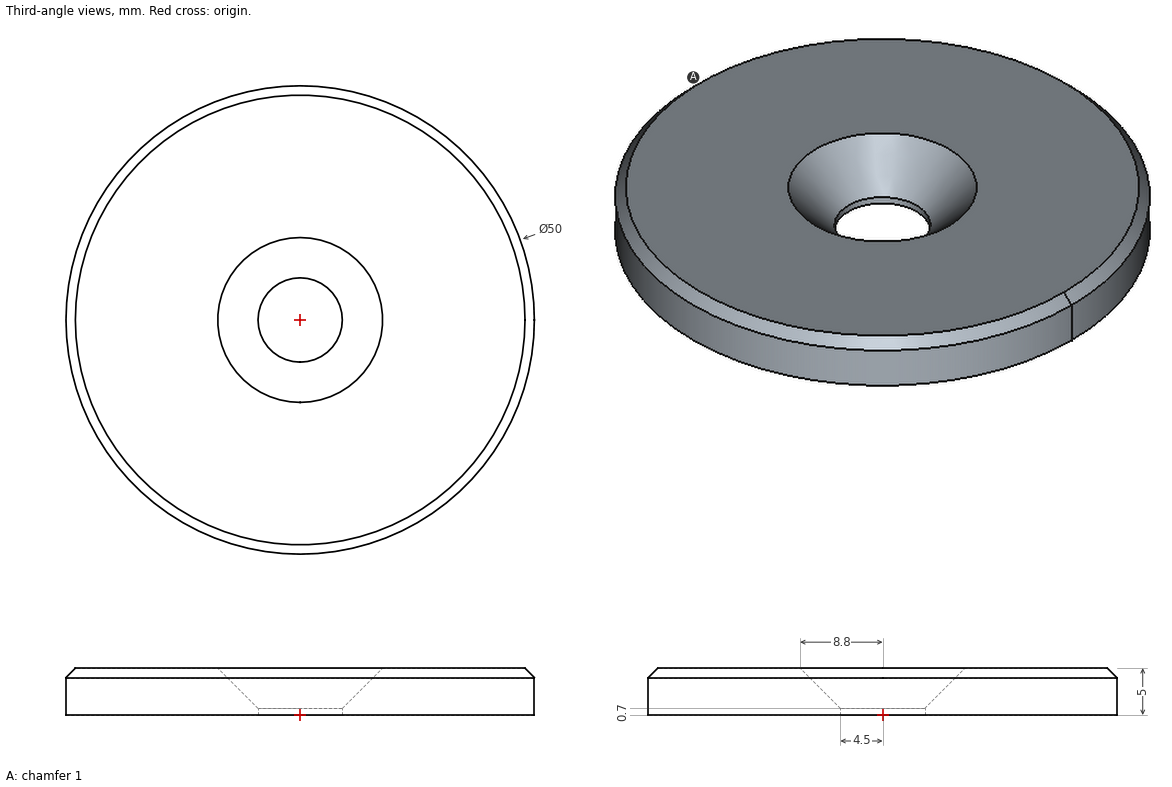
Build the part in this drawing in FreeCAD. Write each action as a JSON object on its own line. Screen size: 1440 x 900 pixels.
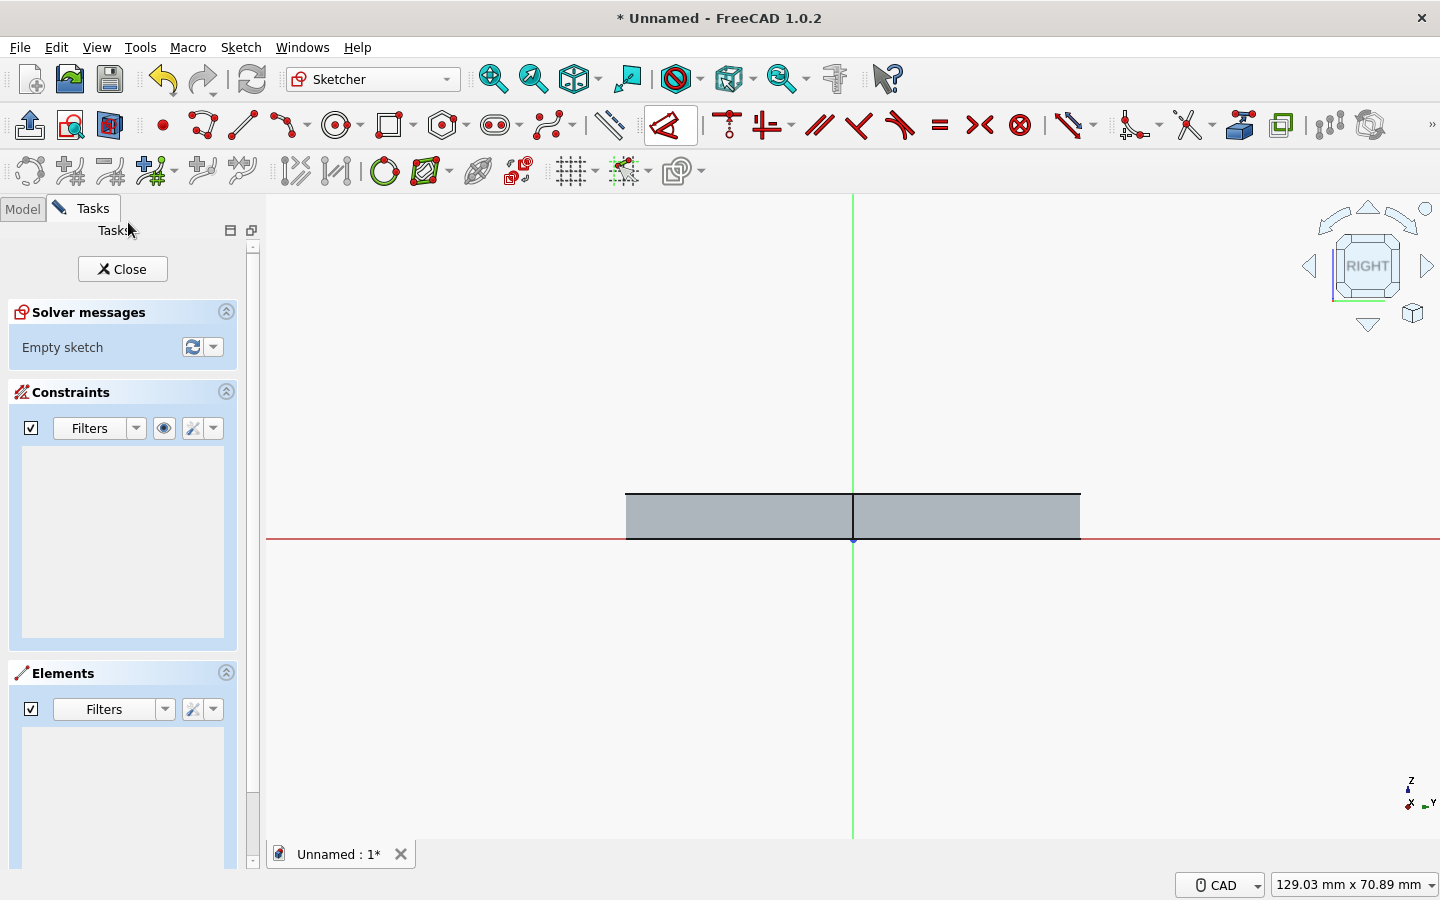
{"action": "left_click", "coordinate": [110, 126]}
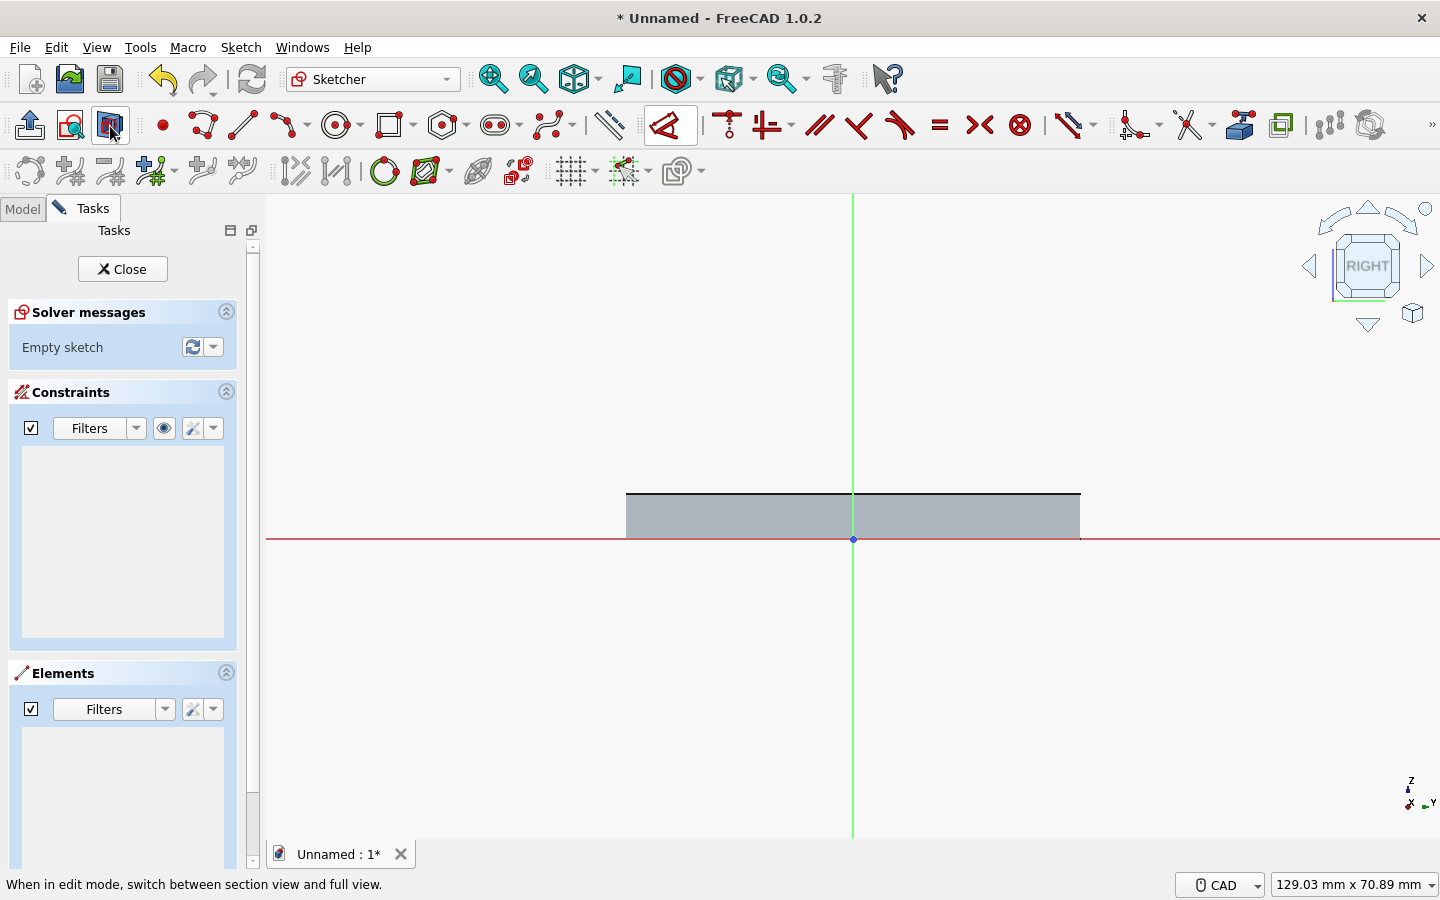
{"action": "scroll", "coordinate": [817, 516], "scroll_direction": "up", "scroll_amount": 11}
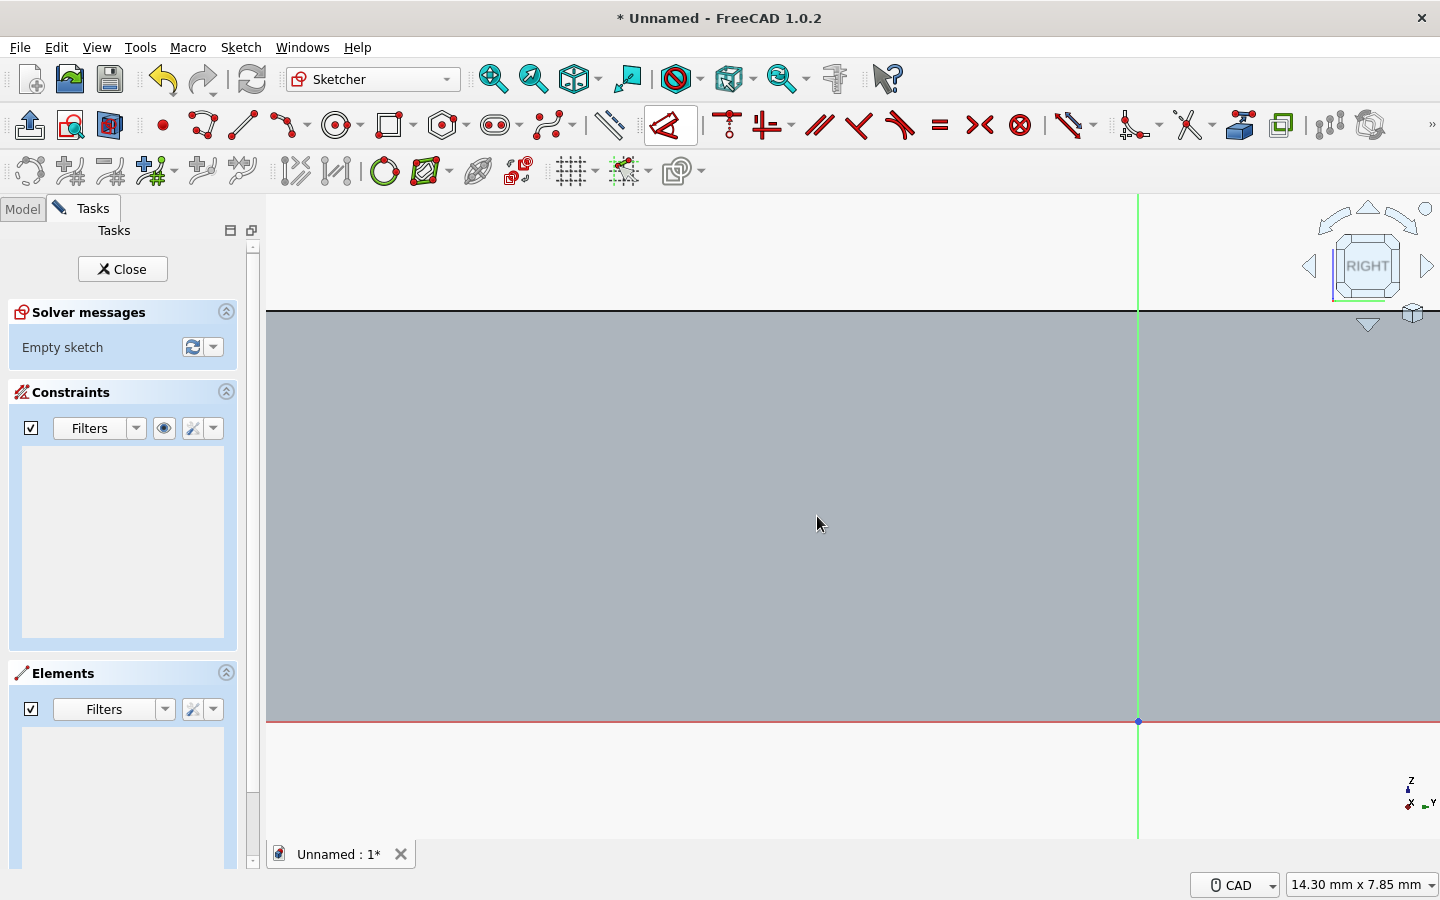
{"action": "left_click", "coordinate": [204, 126]}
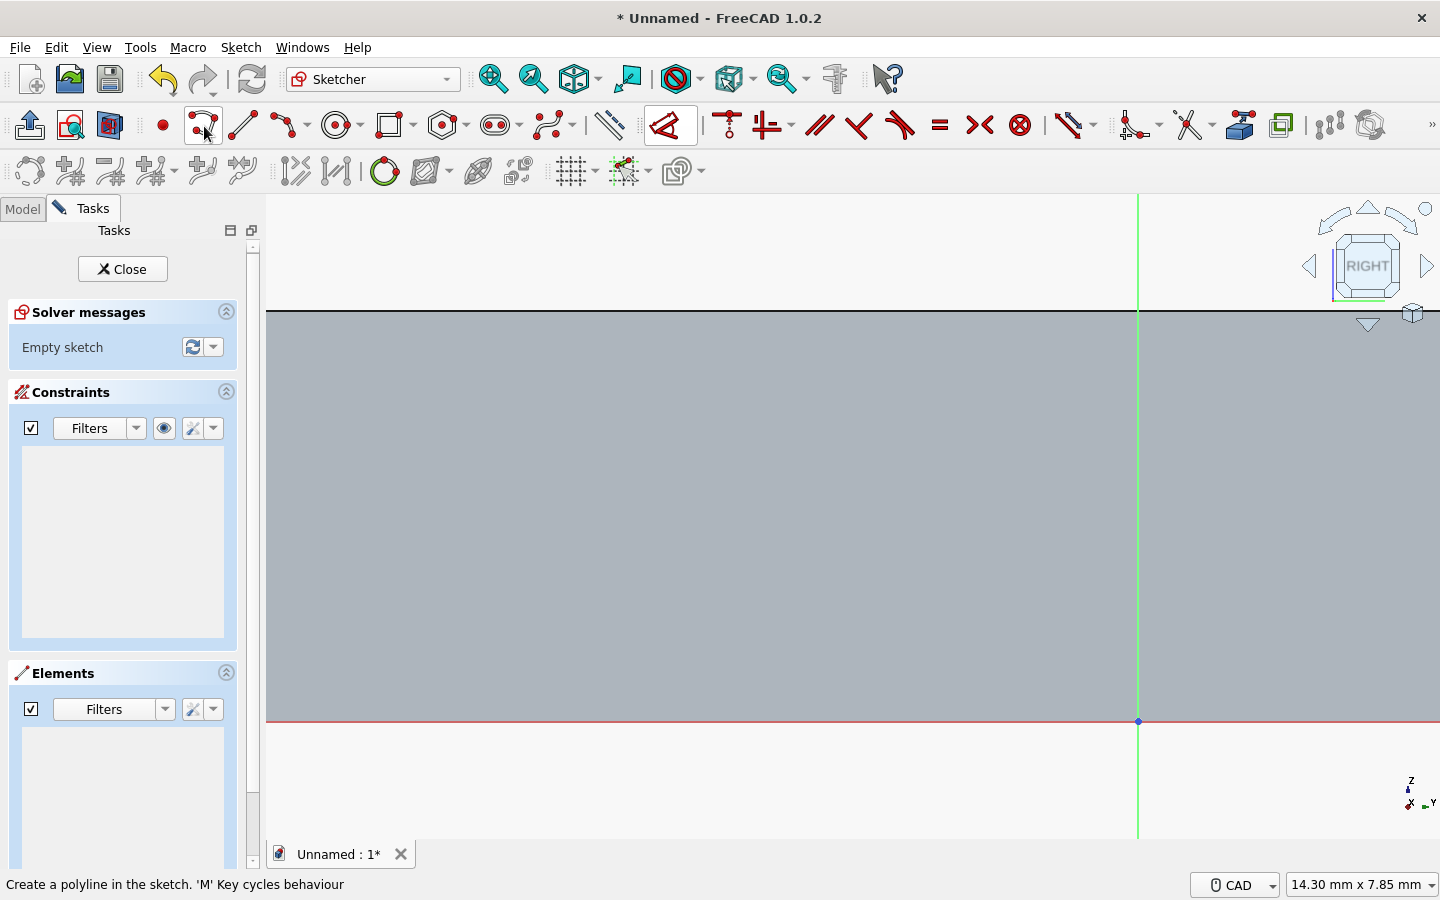
{"action": "left_click", "coordinate": [1138, 722]}
{"action": "left_click", "coordinate": [1129, 311]}
{"action": "left_click", "coordinate": [415, 311]}
{"action": "left_click", "coordinate": [769, 664]}
{"action": "left_click", "coordinate": [769, 713]}
{"action": "left_click", "coordinate": [1138, 722]}
{"action": "key", "text": "Escape"}
{"action": "key", "text": "Escape"}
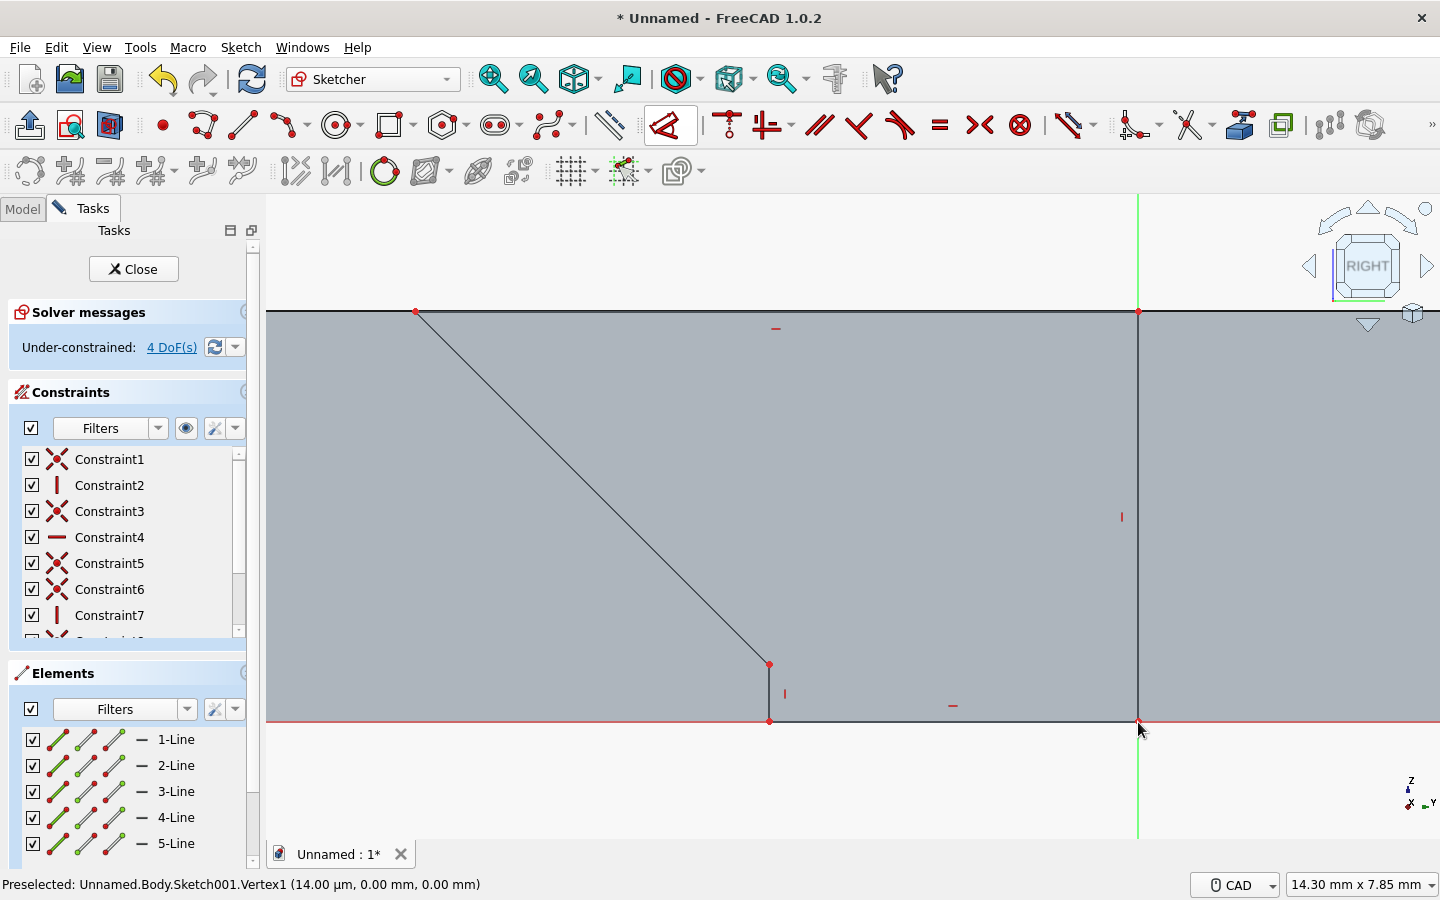
{"action": "left_click", "coordinate": [664, 126]}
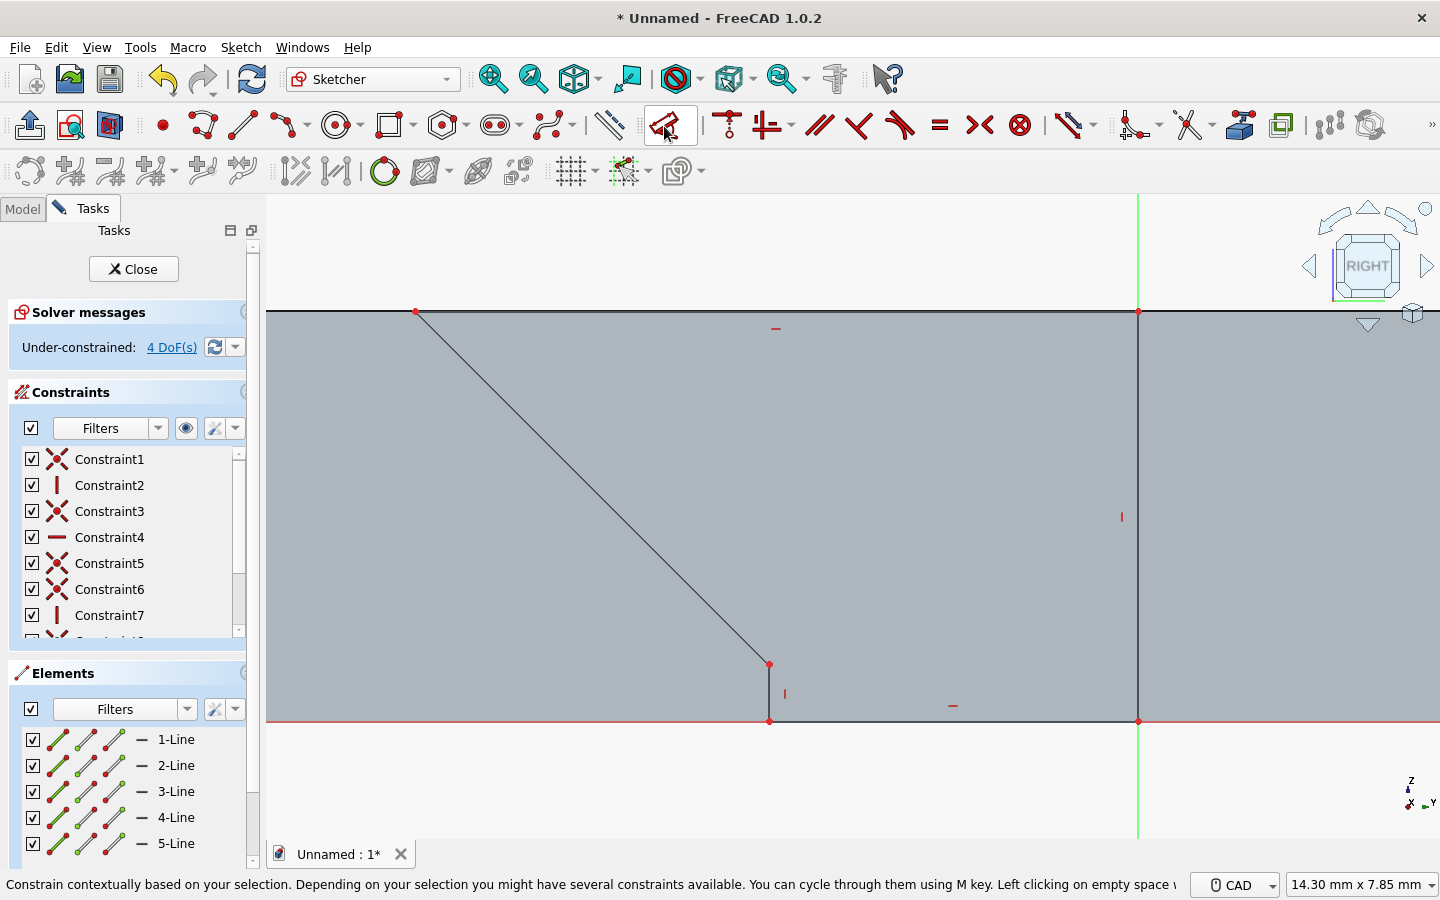
{"action": "left_click", "coordinate": [1138, 599]}
{"action": "left_click", "coordinate": [1172, 517]}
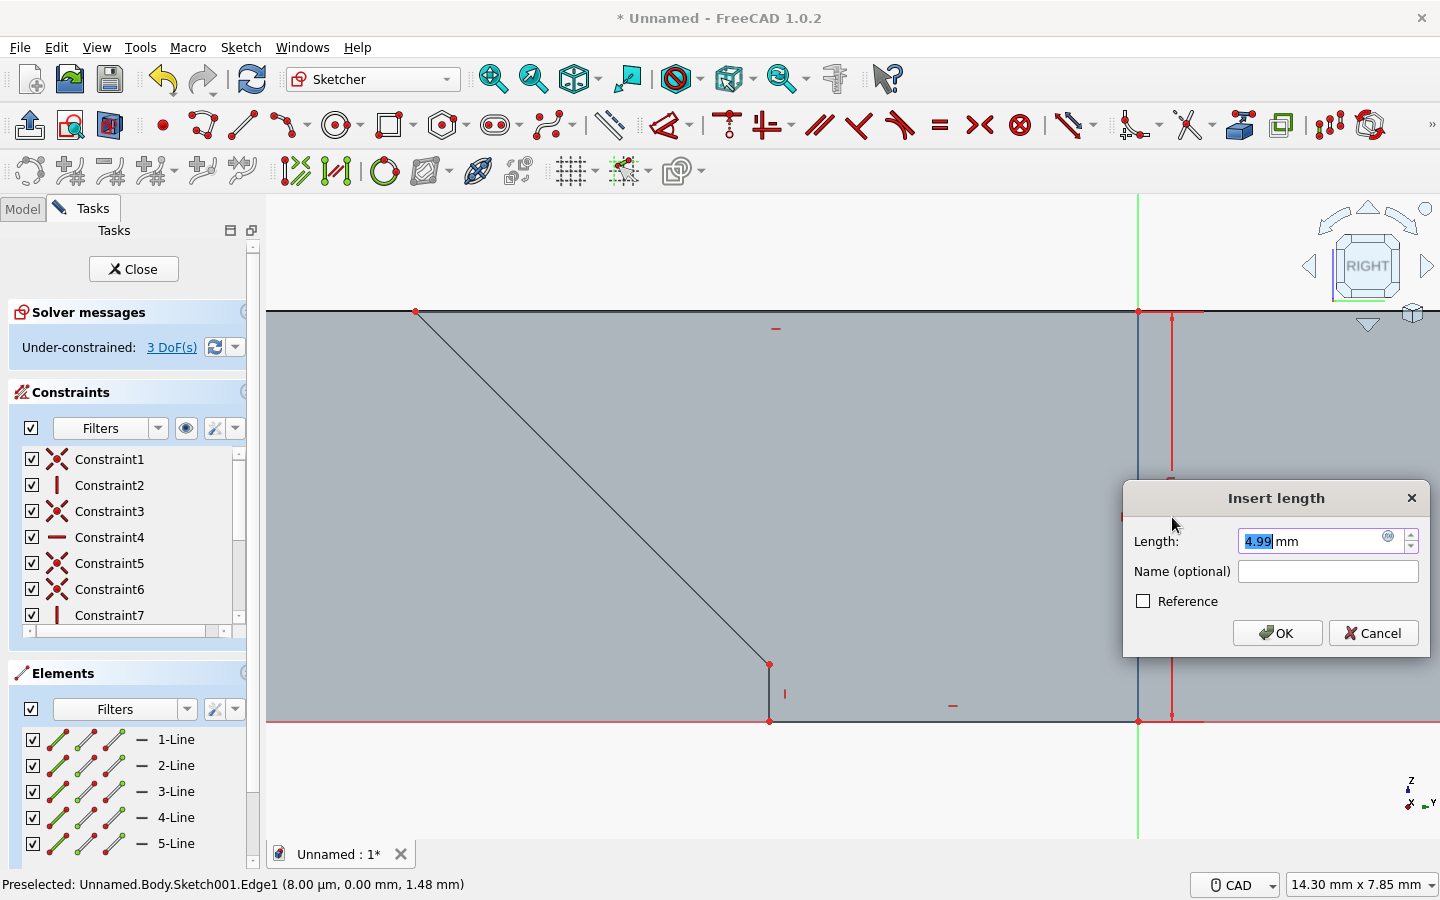
{"action": "type", "text": "5"}
{"action": "key", "text": "Return"}